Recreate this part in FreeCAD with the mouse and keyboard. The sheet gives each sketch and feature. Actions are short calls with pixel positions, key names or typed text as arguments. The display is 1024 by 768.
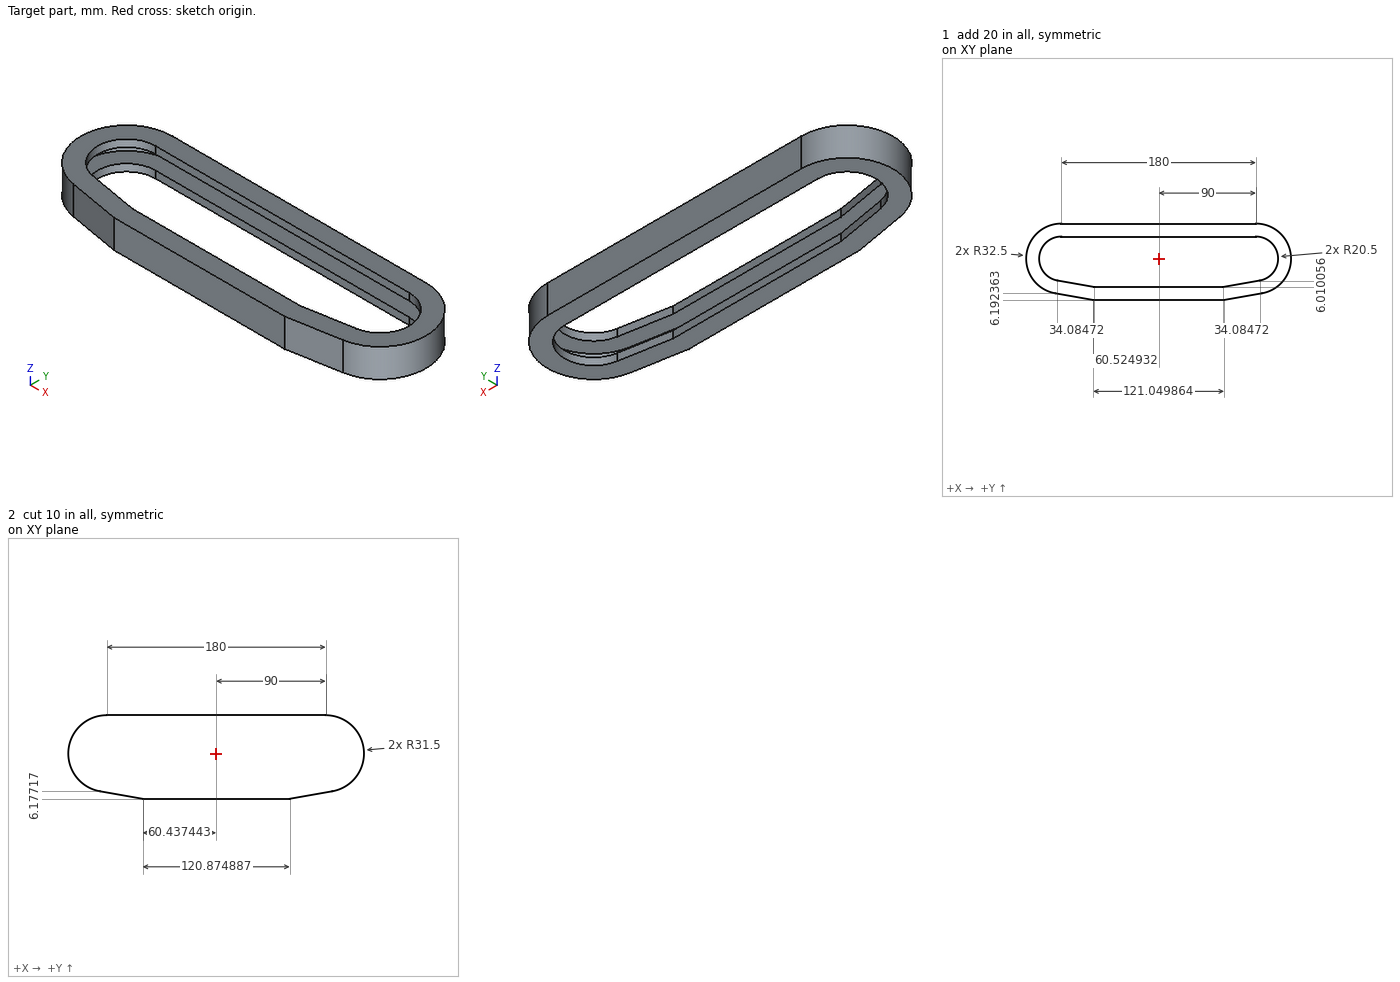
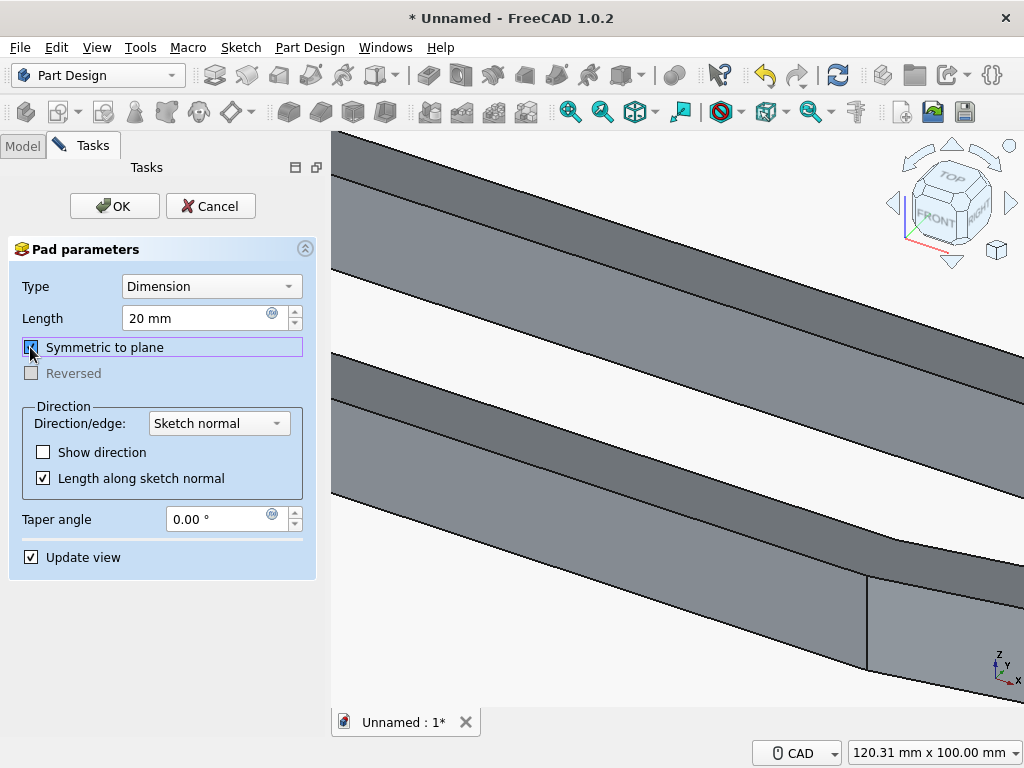
click(115, 206)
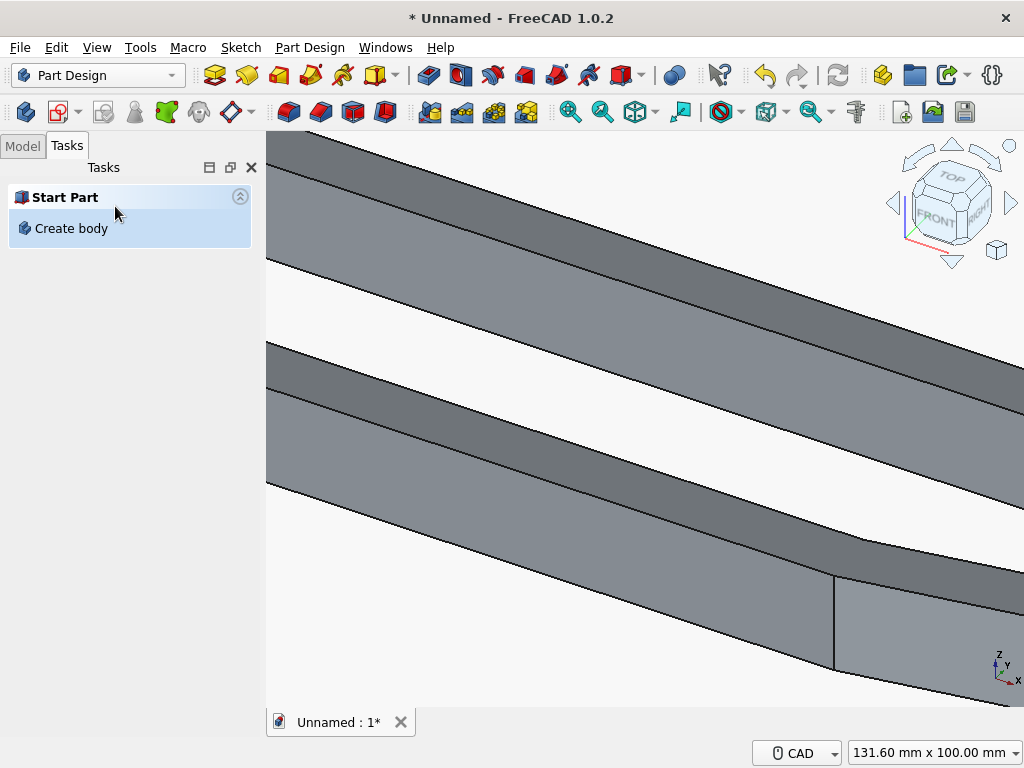
click(572, 112)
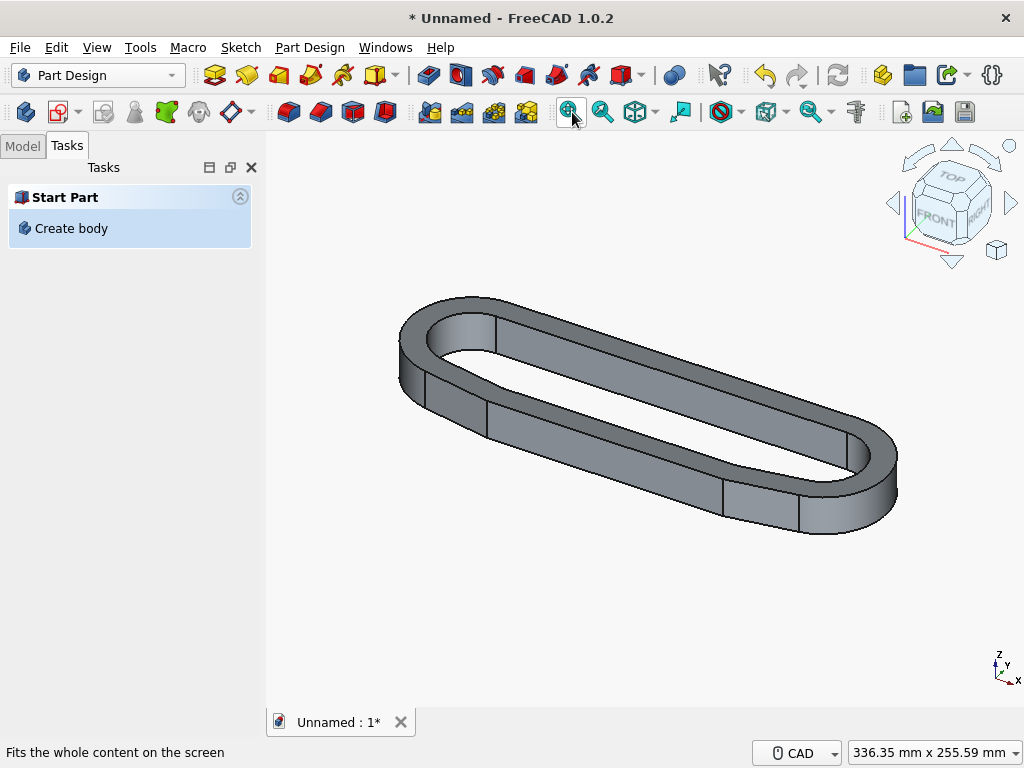
click(58, 112)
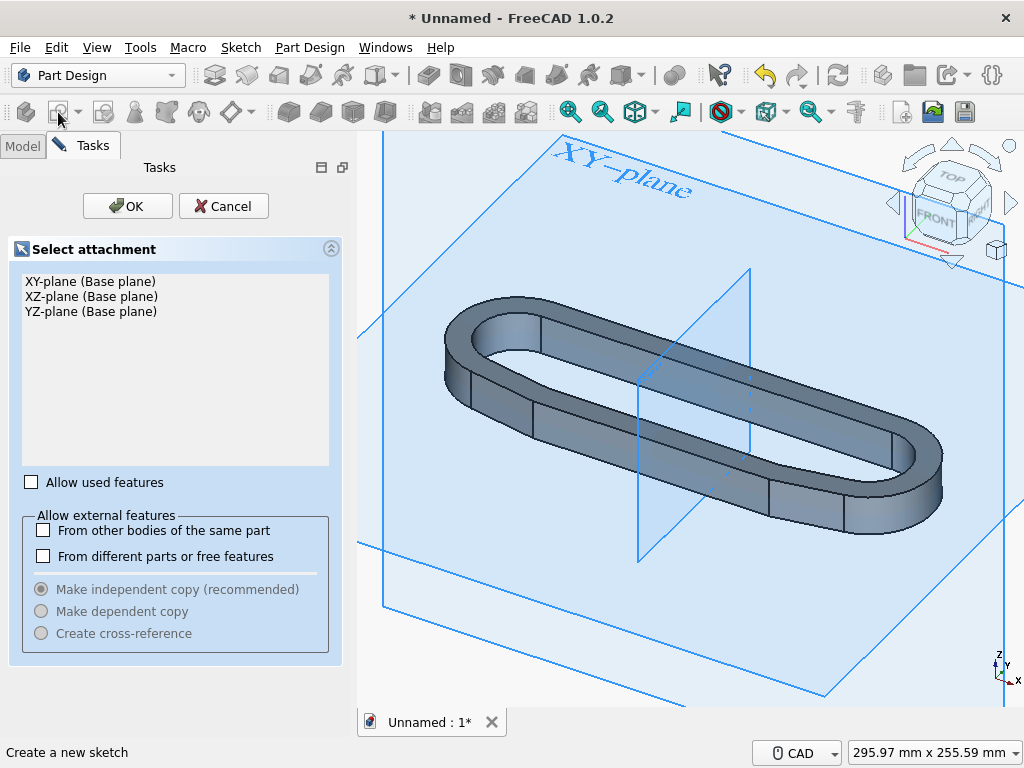
click(82, 282)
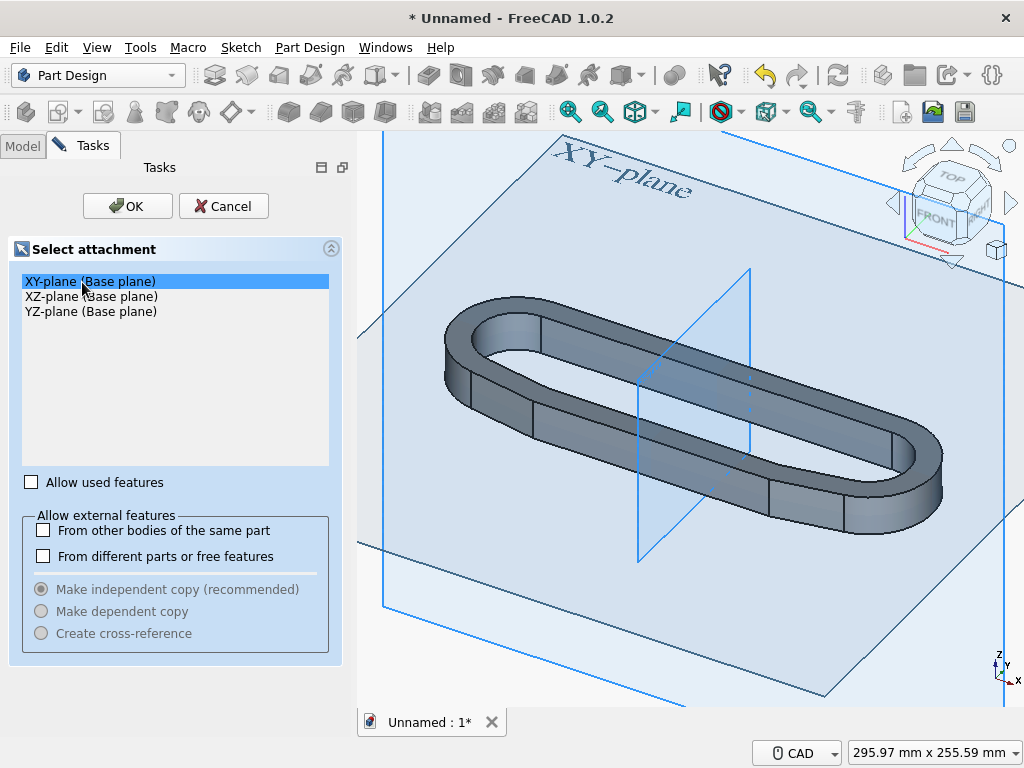
click(128, 206)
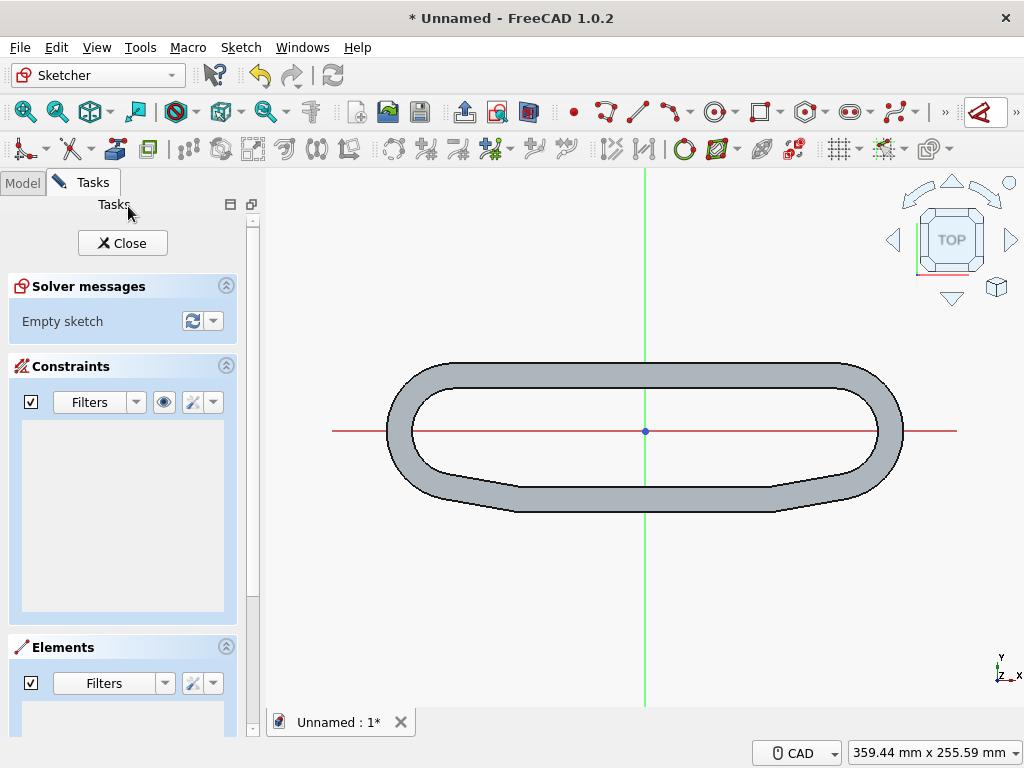
click(530, 112)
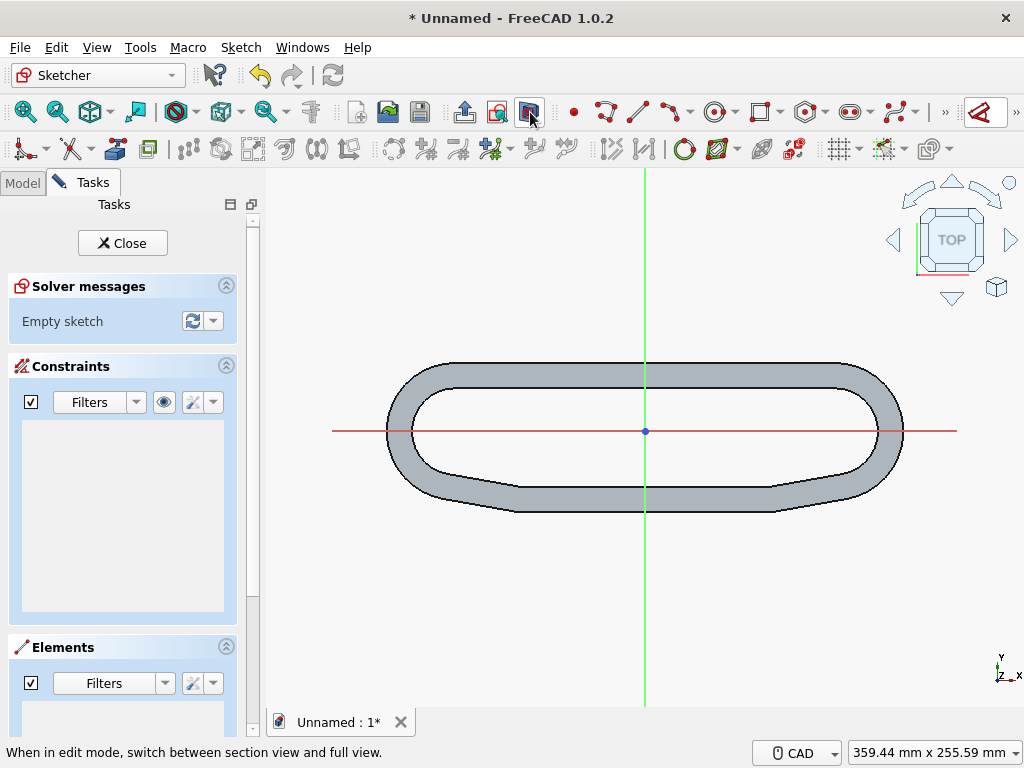
scroll(294, 438, down, 1)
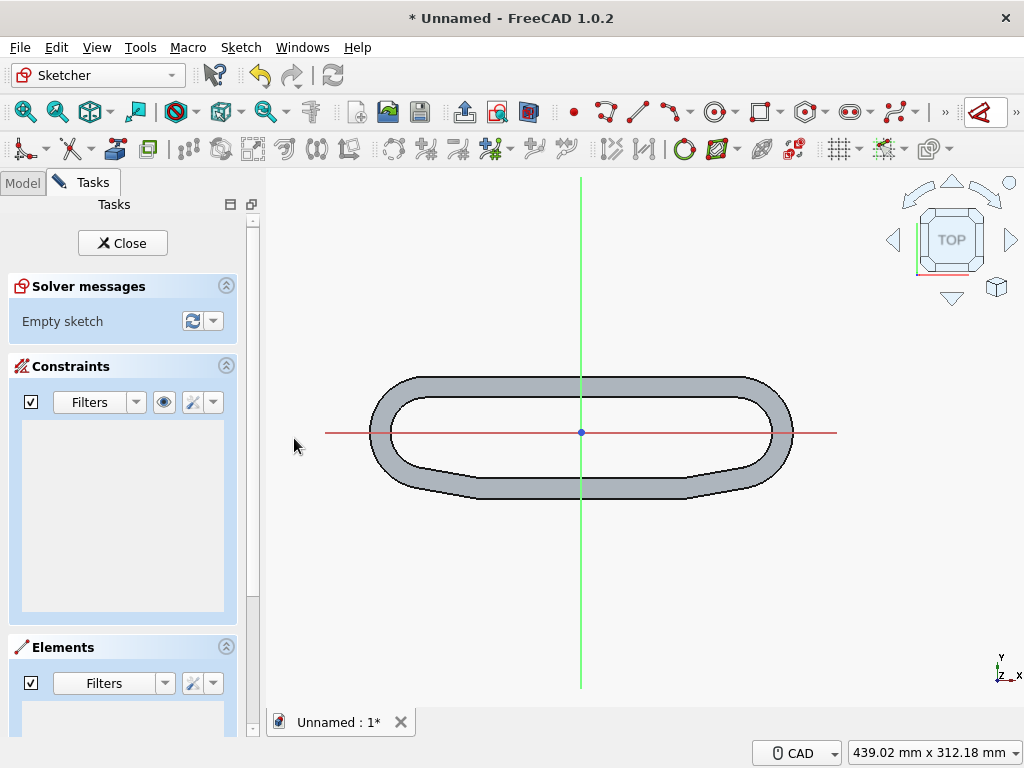
click(638, 112)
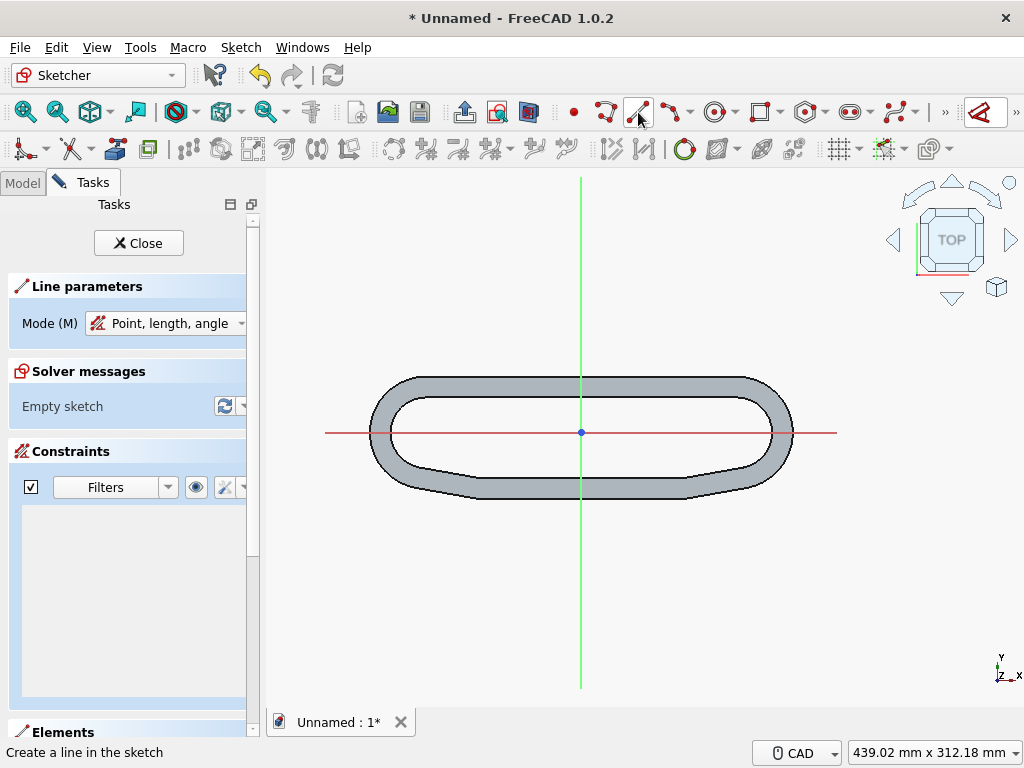
click(737, 378)
click(426, 378)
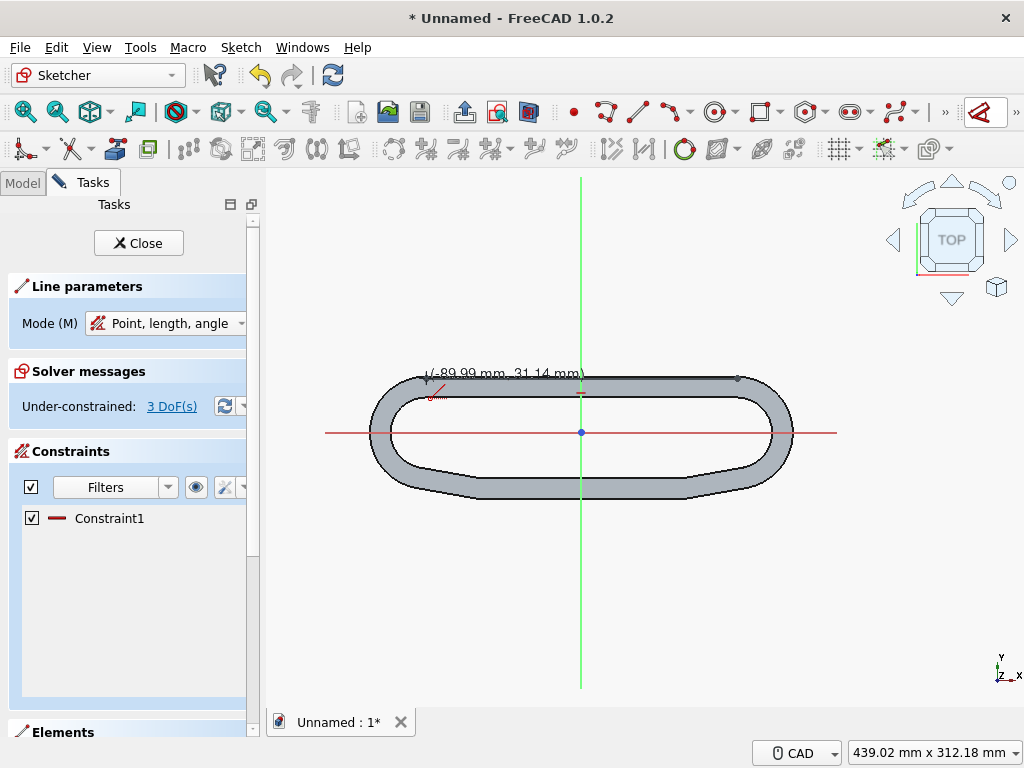
click(606, 112)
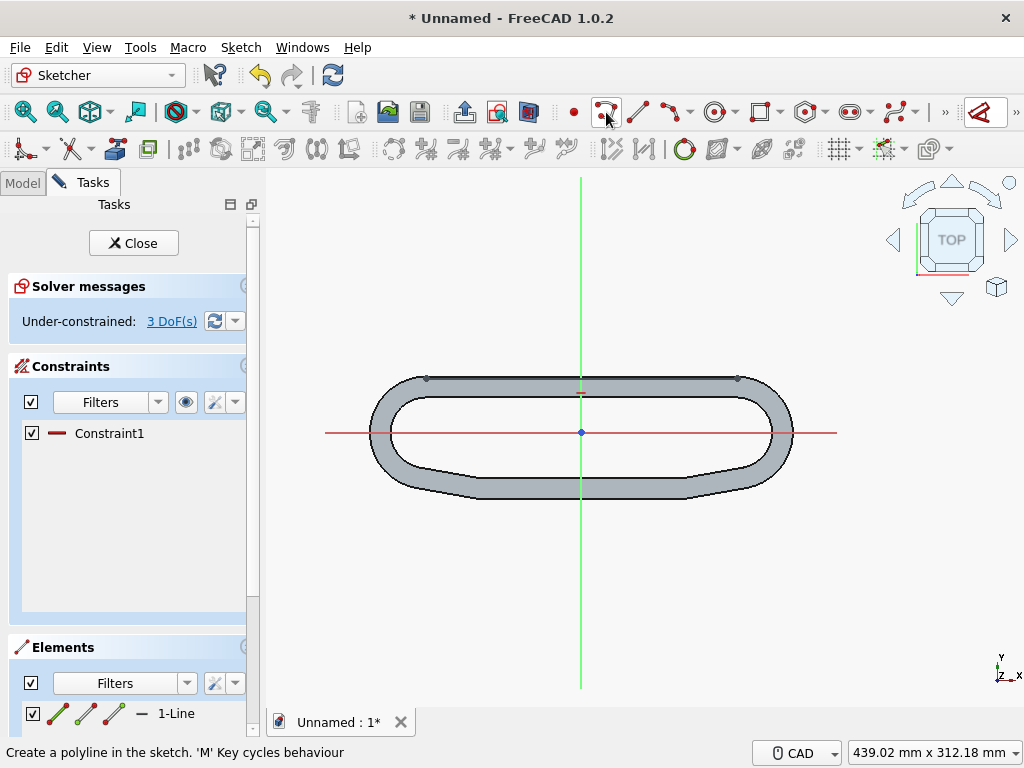
click(417, 486)
click(477, 497)
click(686, 497)
click(746, 486)
right_click(746, 486)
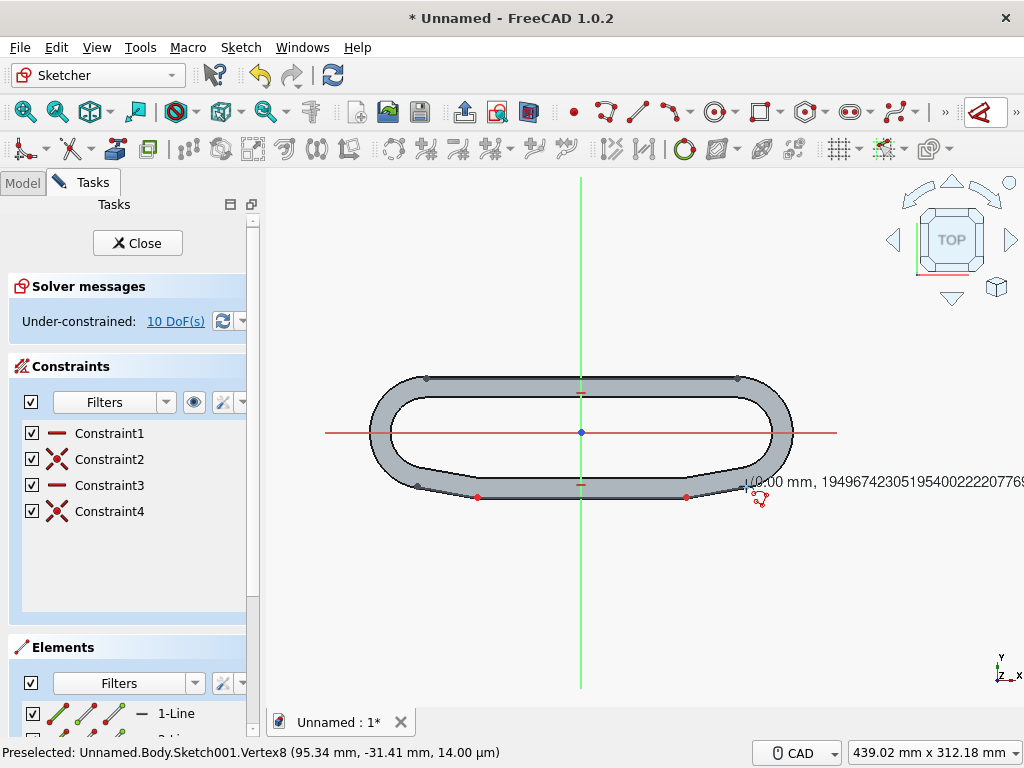
key(g)
key(3)
key(a)